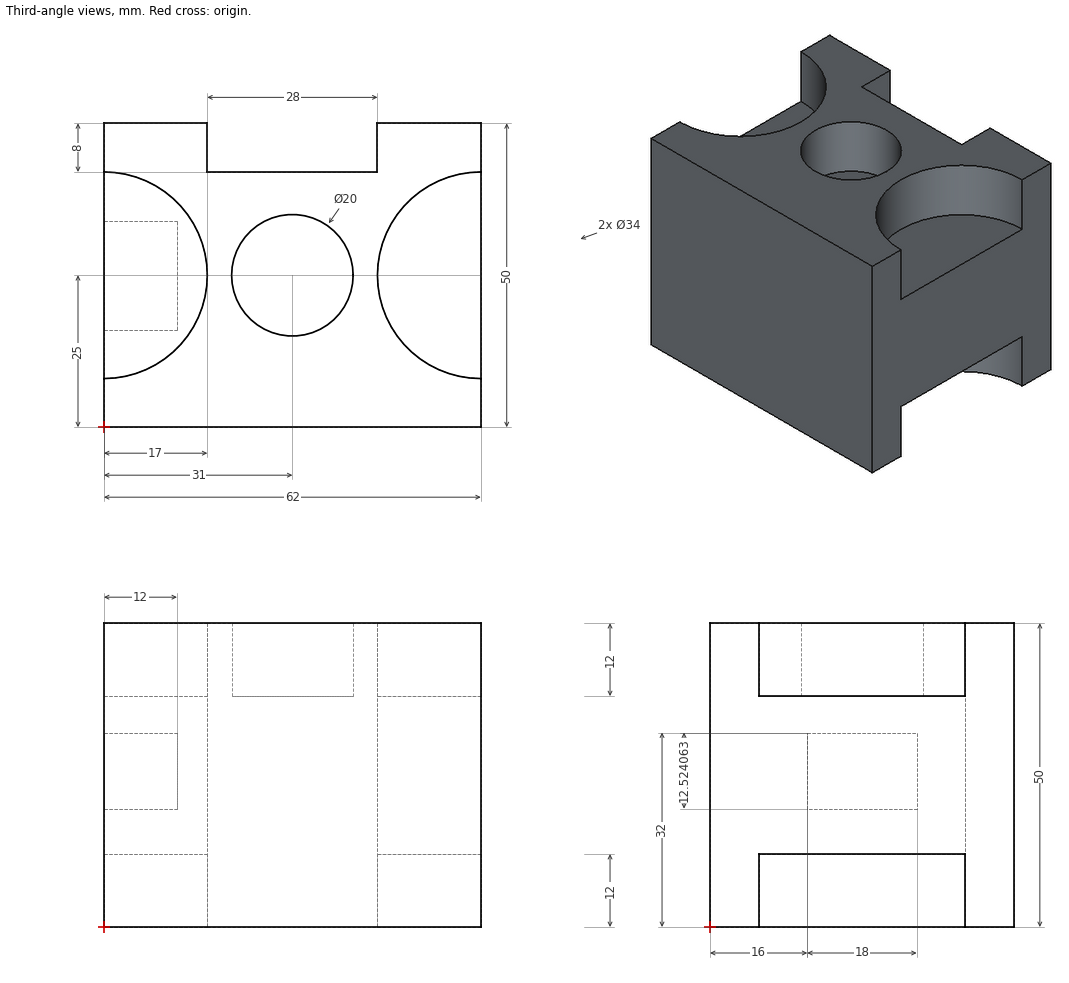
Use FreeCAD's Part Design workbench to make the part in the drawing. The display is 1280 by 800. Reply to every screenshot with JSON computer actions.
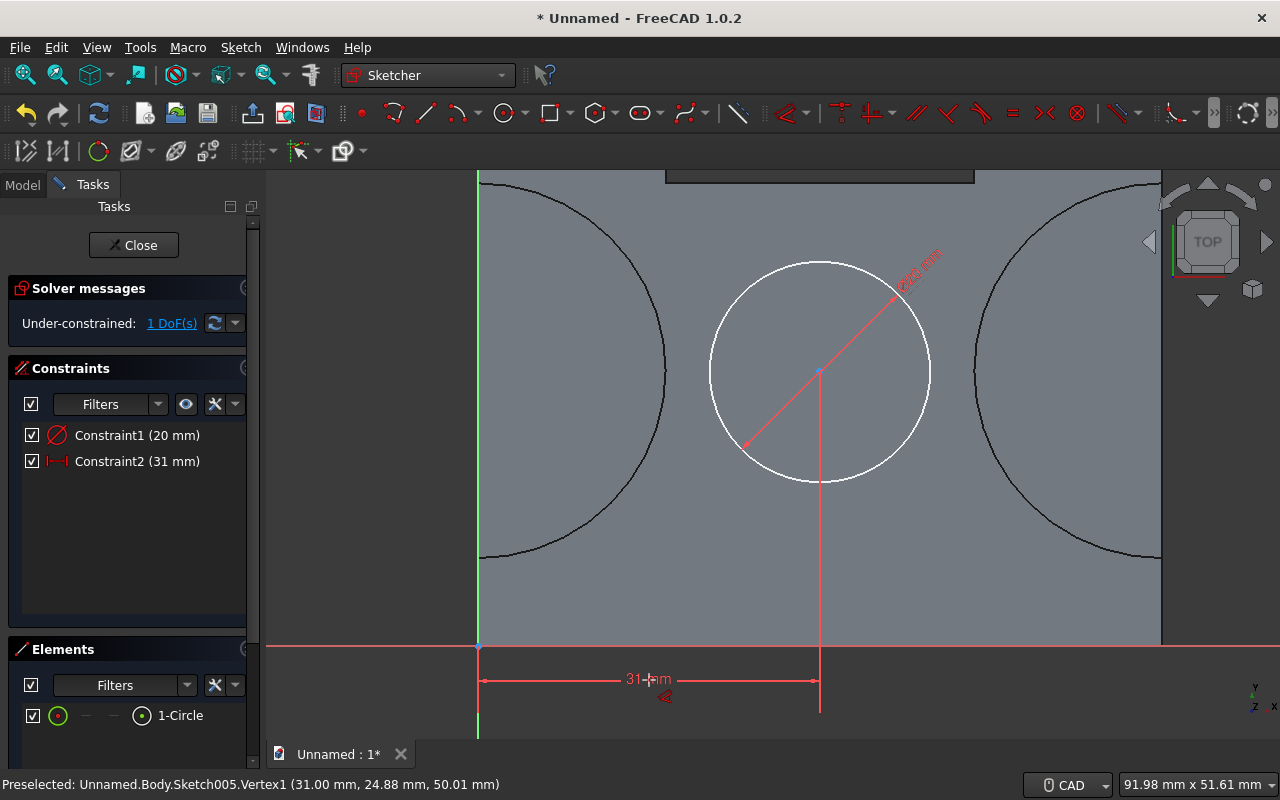
{"action": "left_click", "coordinate": [820, 372]}
{"action": "left_click", "coordinate": [444, 509]}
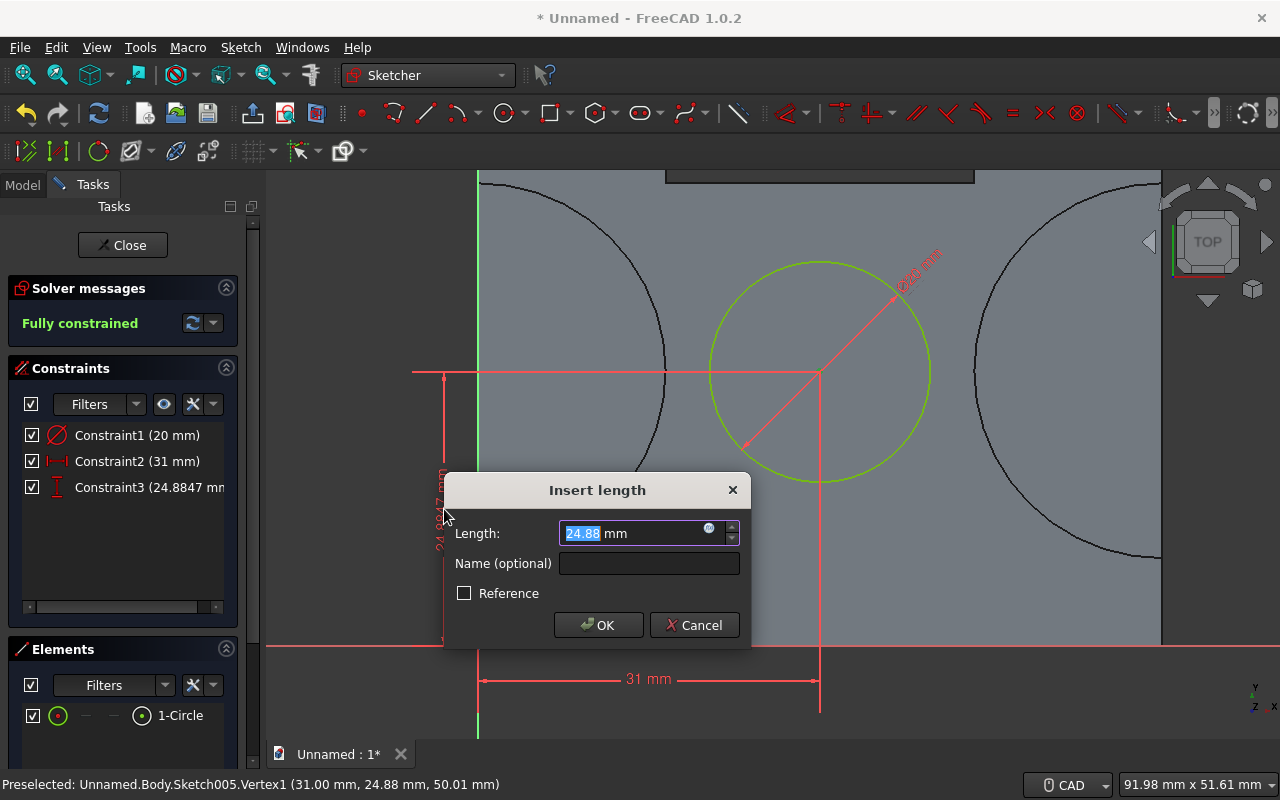
{"action": "type", "text": "25"}
{"action": "key", "text": "Return"}
{"action": "key", "text": "Escape"}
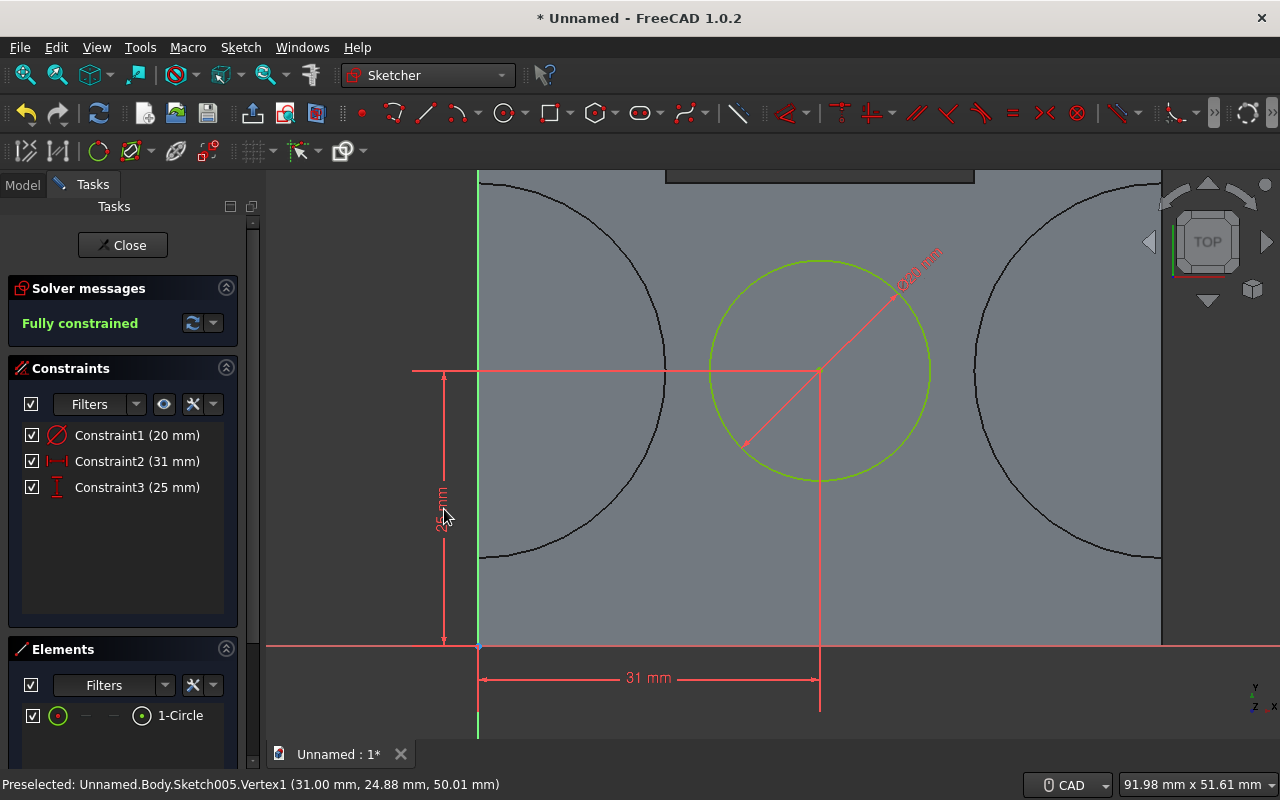
{"action": "left_click", "coordinate": [123, 245]}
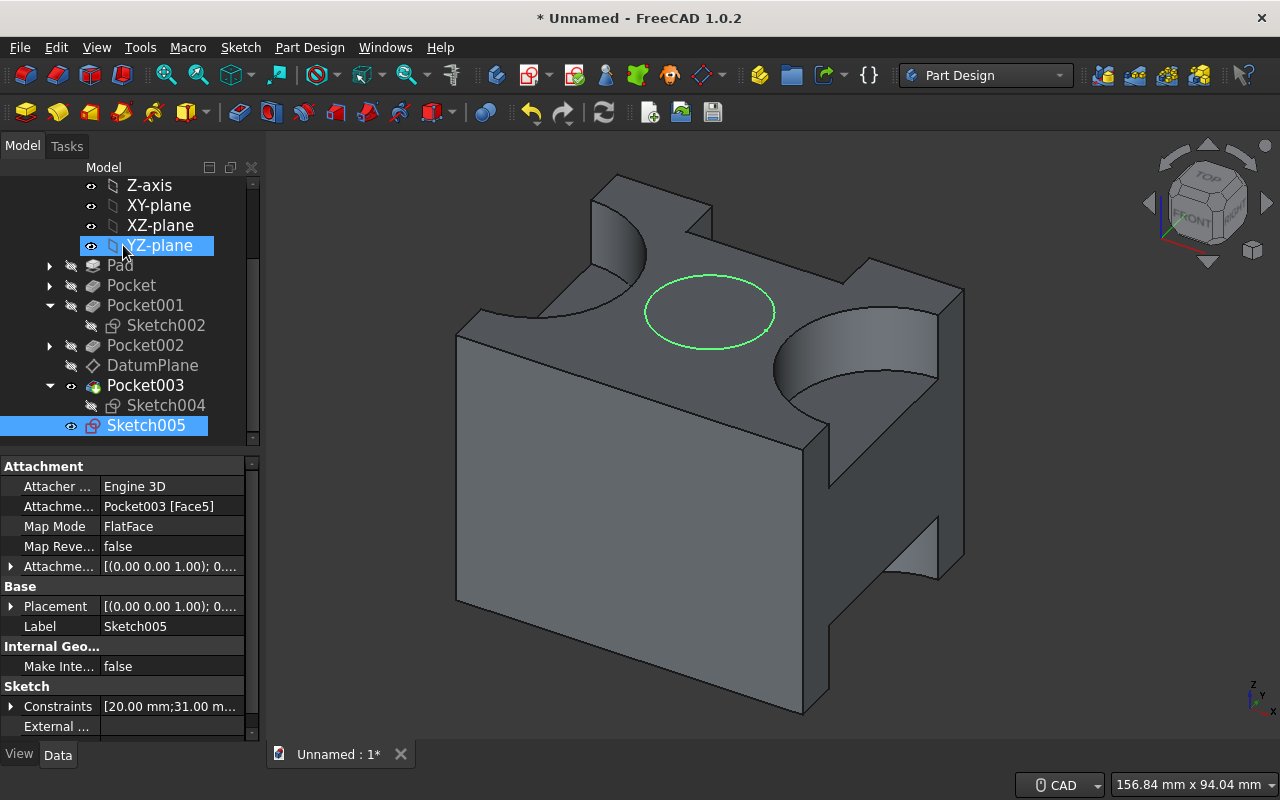
{"action": "left_click", "coordinate": [240, 112]}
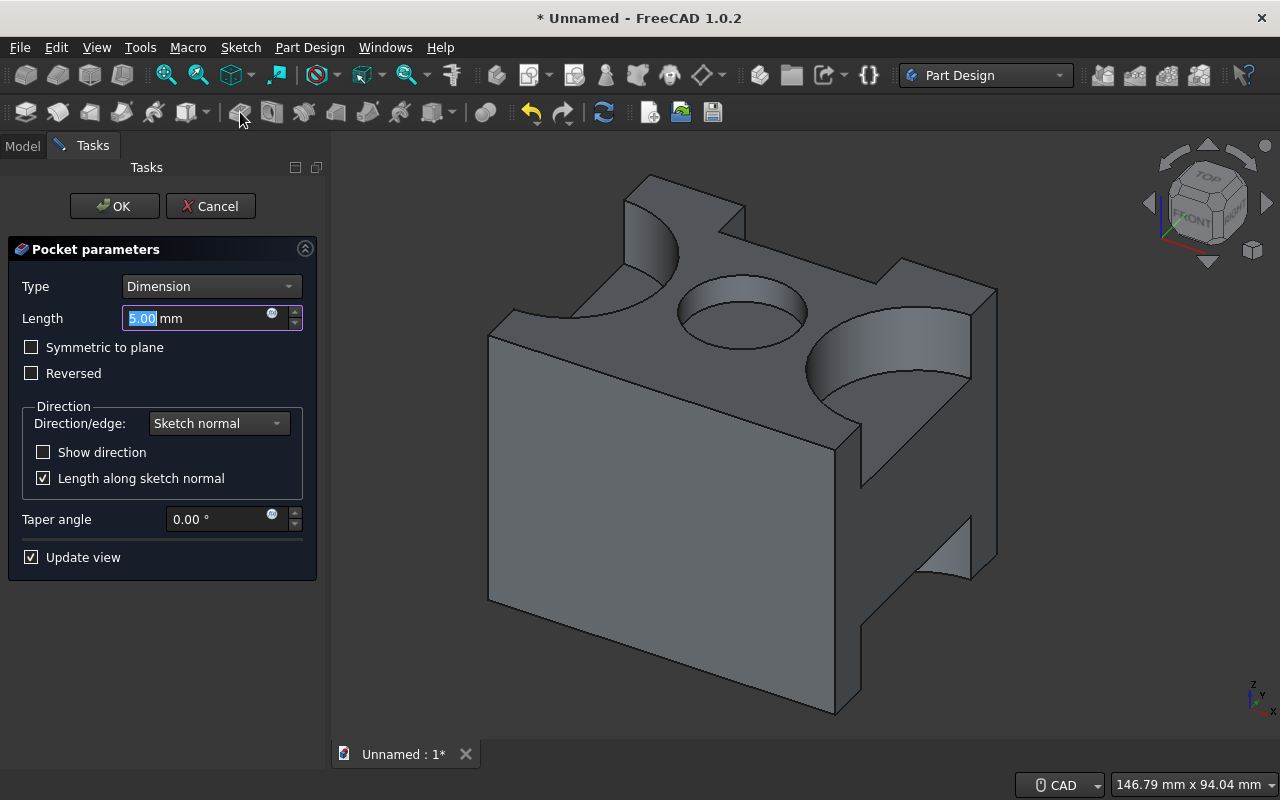
{"action": "type", "text": "12"}
{"action": "key", "text": "Tab"}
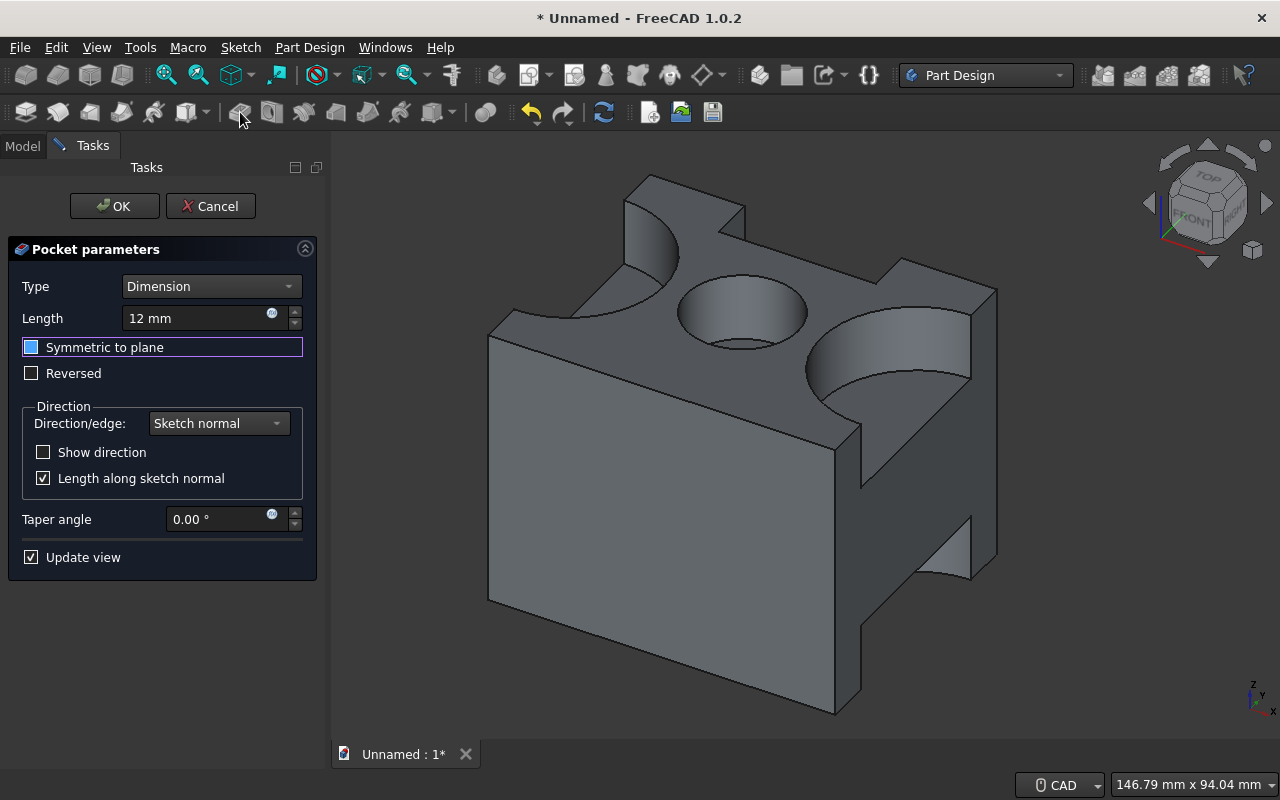
{"action": "left_click", "coordinate": [115, 206]}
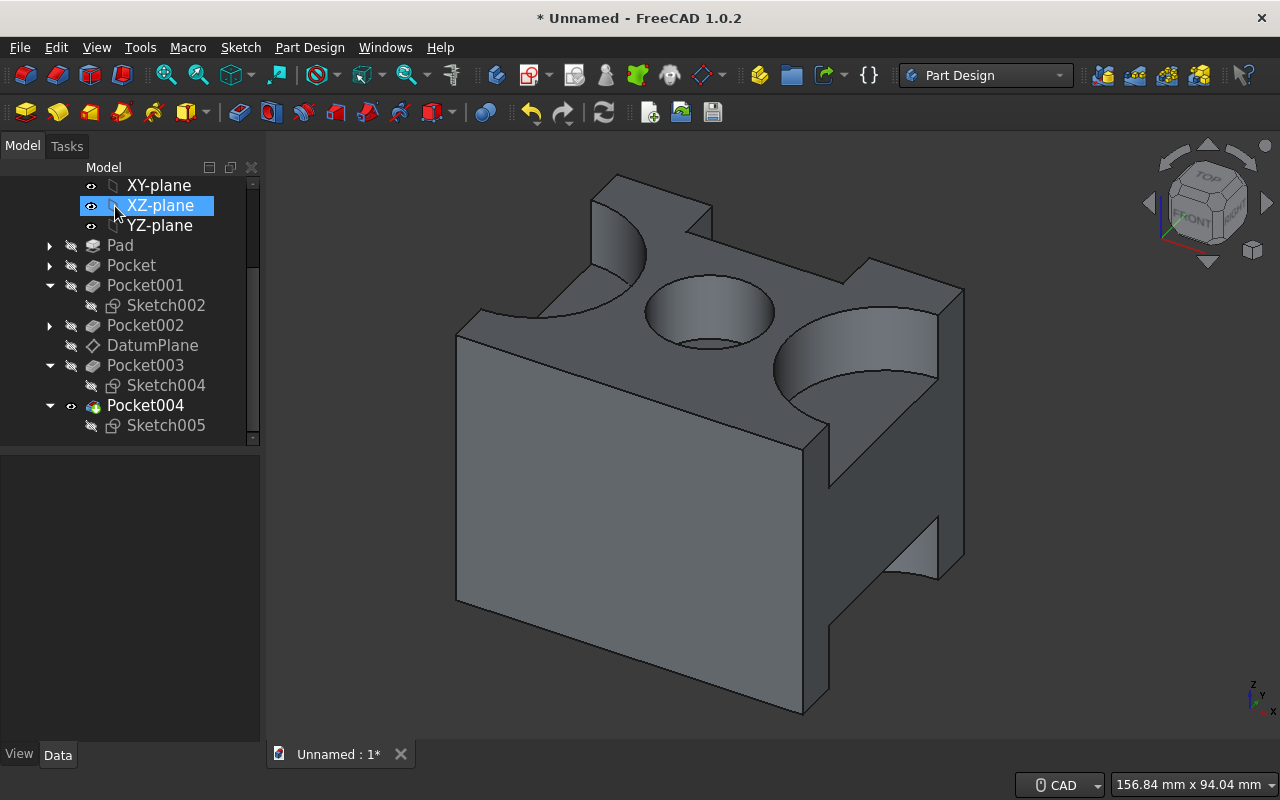
{"action": "key", "text": "0"}